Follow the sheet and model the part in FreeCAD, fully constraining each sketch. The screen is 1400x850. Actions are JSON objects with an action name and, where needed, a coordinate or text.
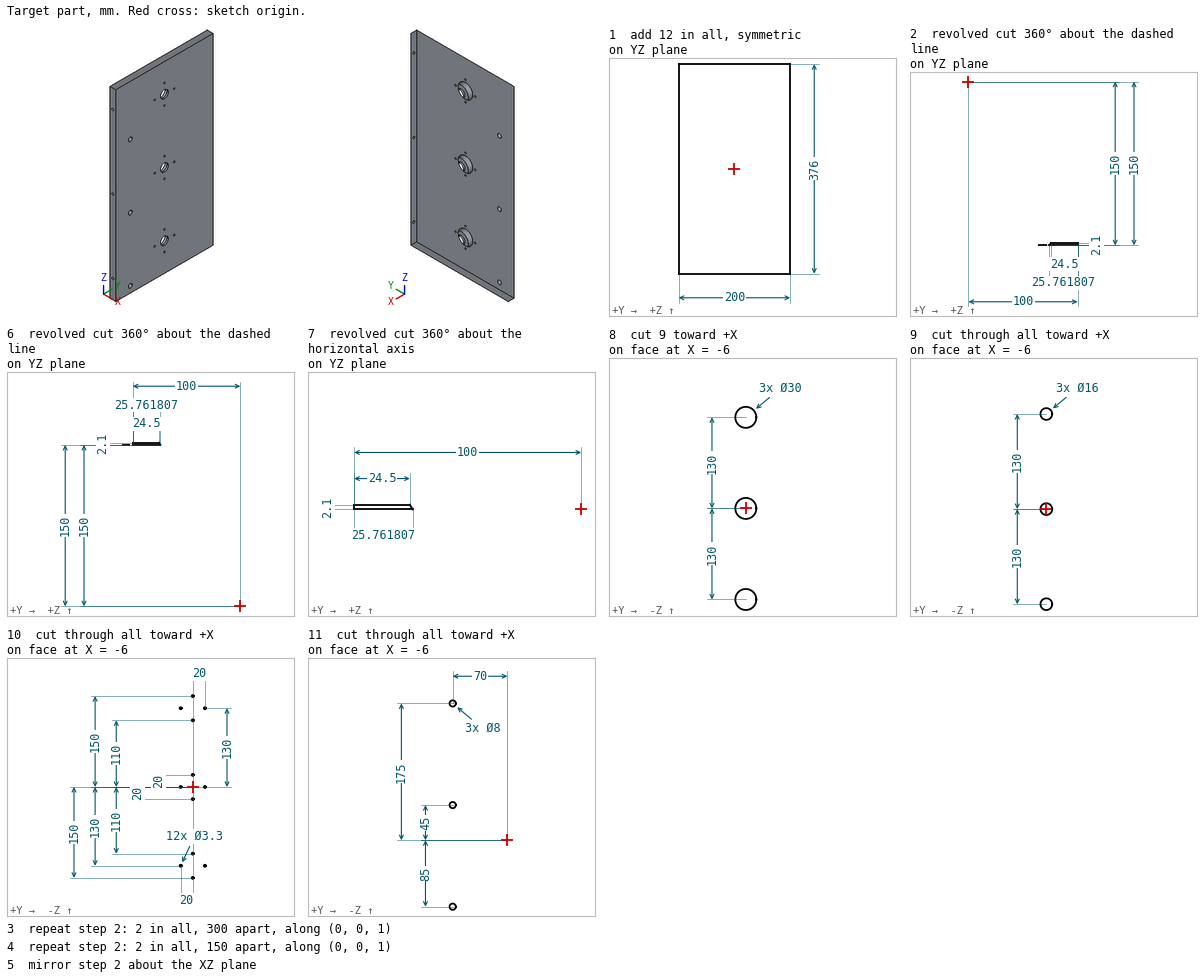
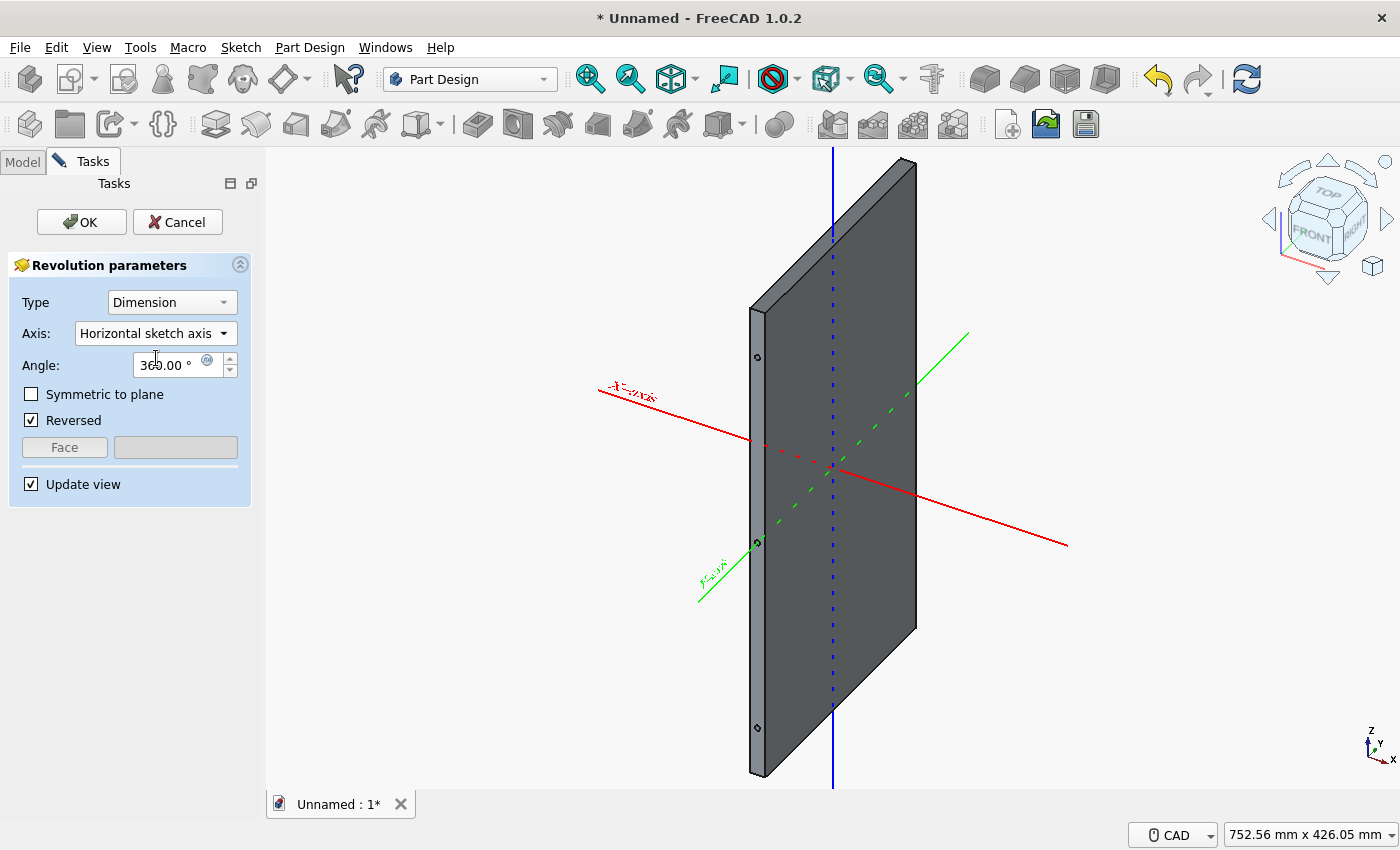
{"action": "left_click", "coordinate": [82, 222]}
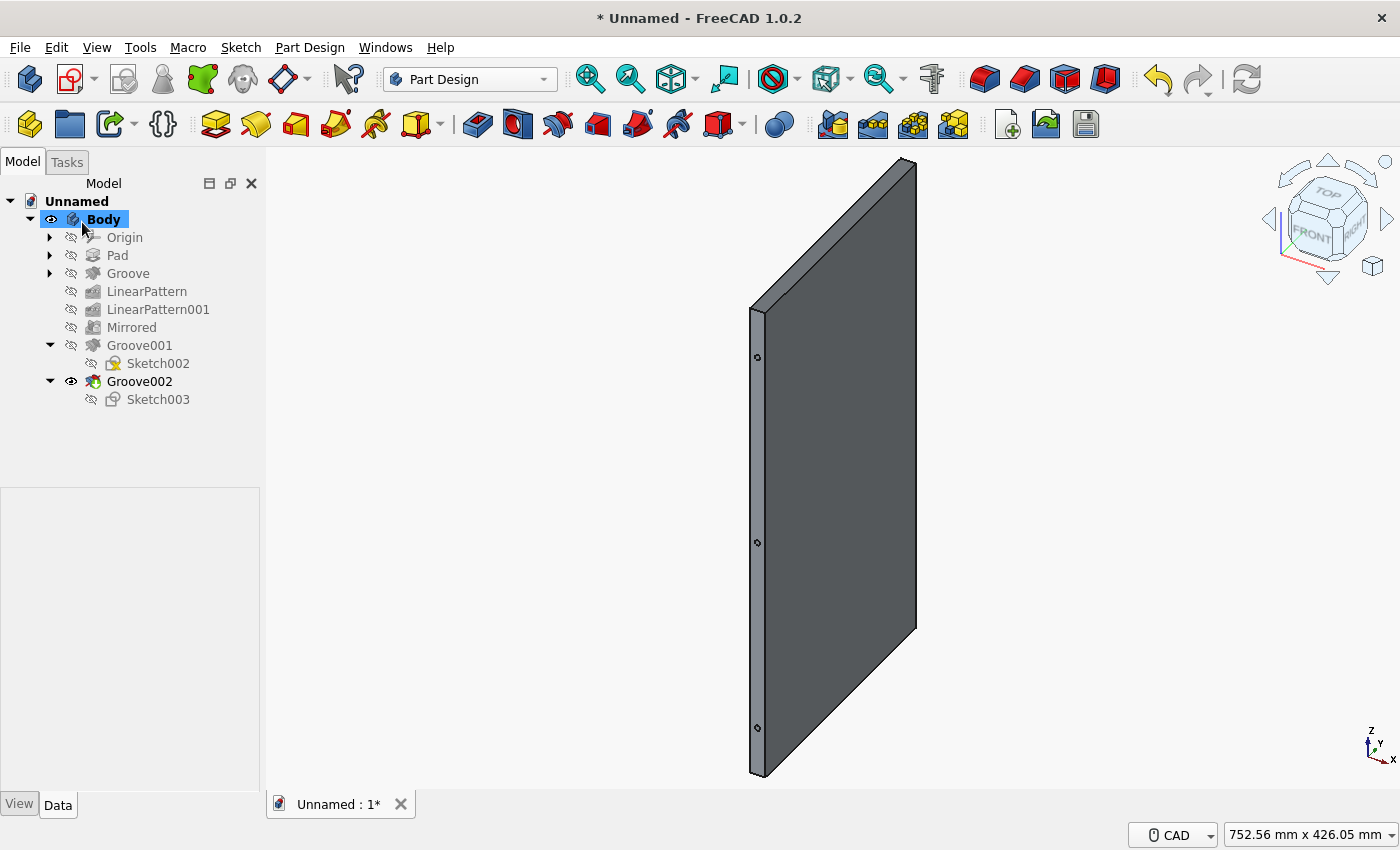
{"action": "key", "text": "6"}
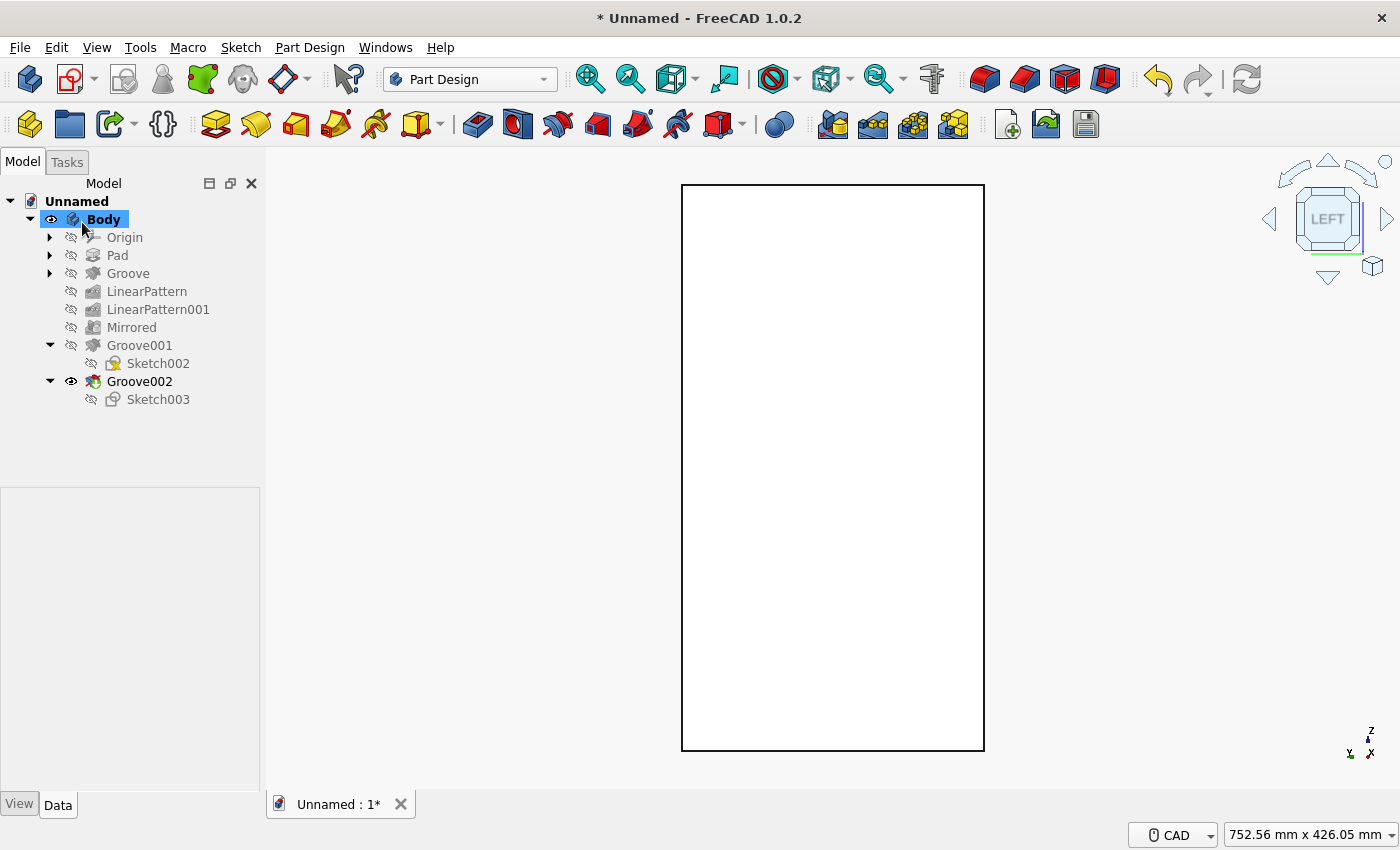
{"action": "left_click", "coordinate": [833, 467]}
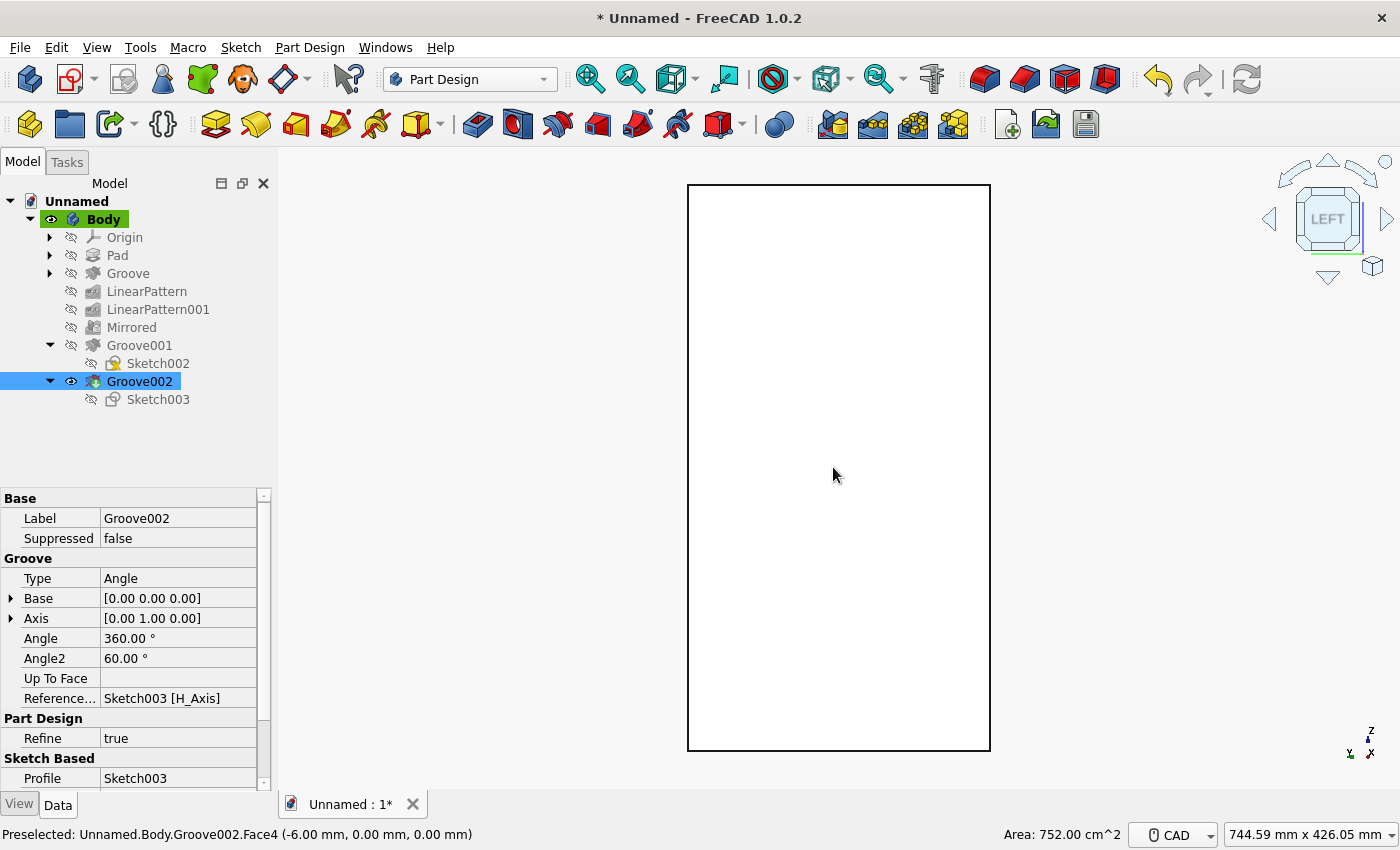
{"action": "left_click", "coordinate": [70, 80]}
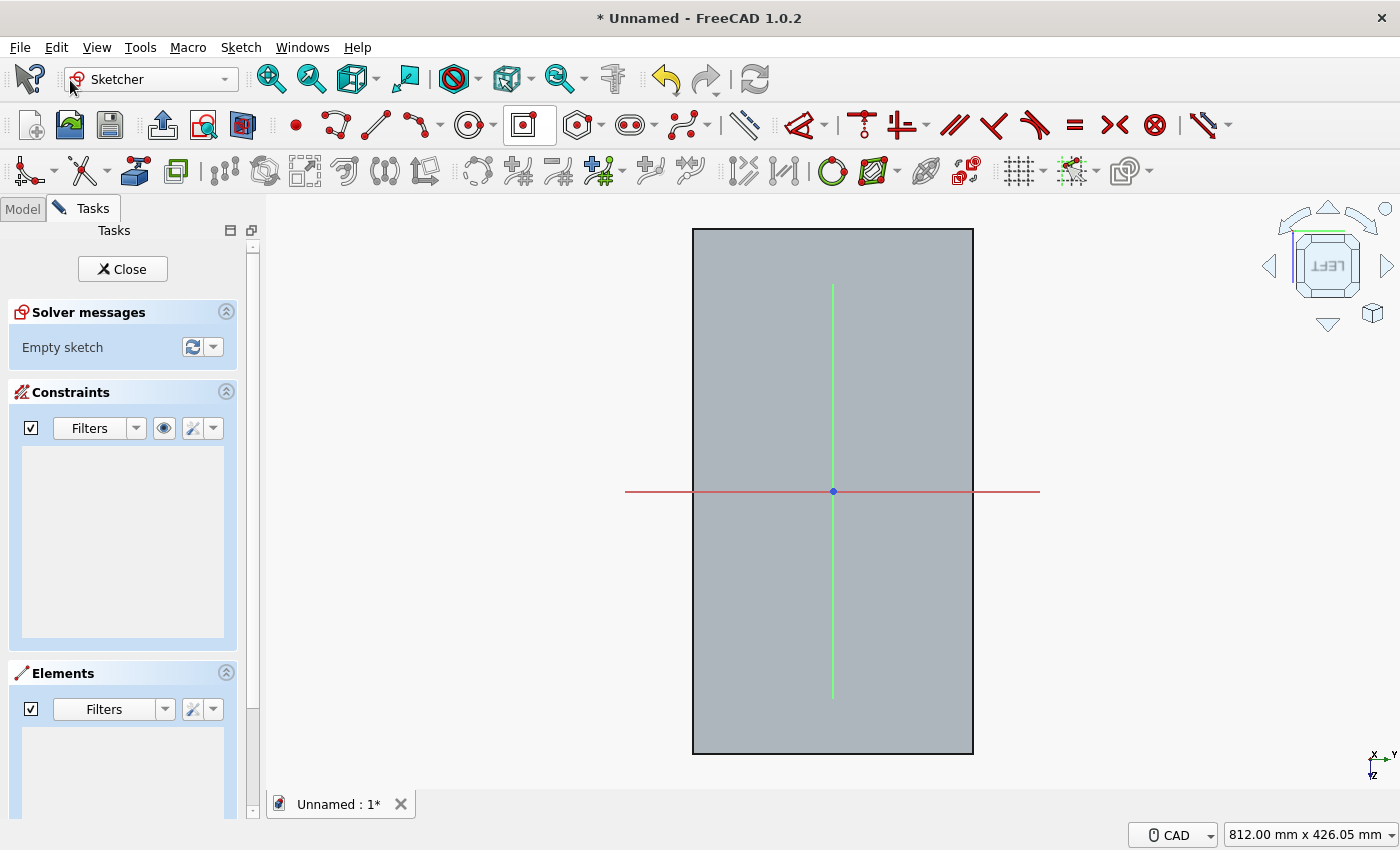
{"action": "left_click", "coordinate": [470, 126]}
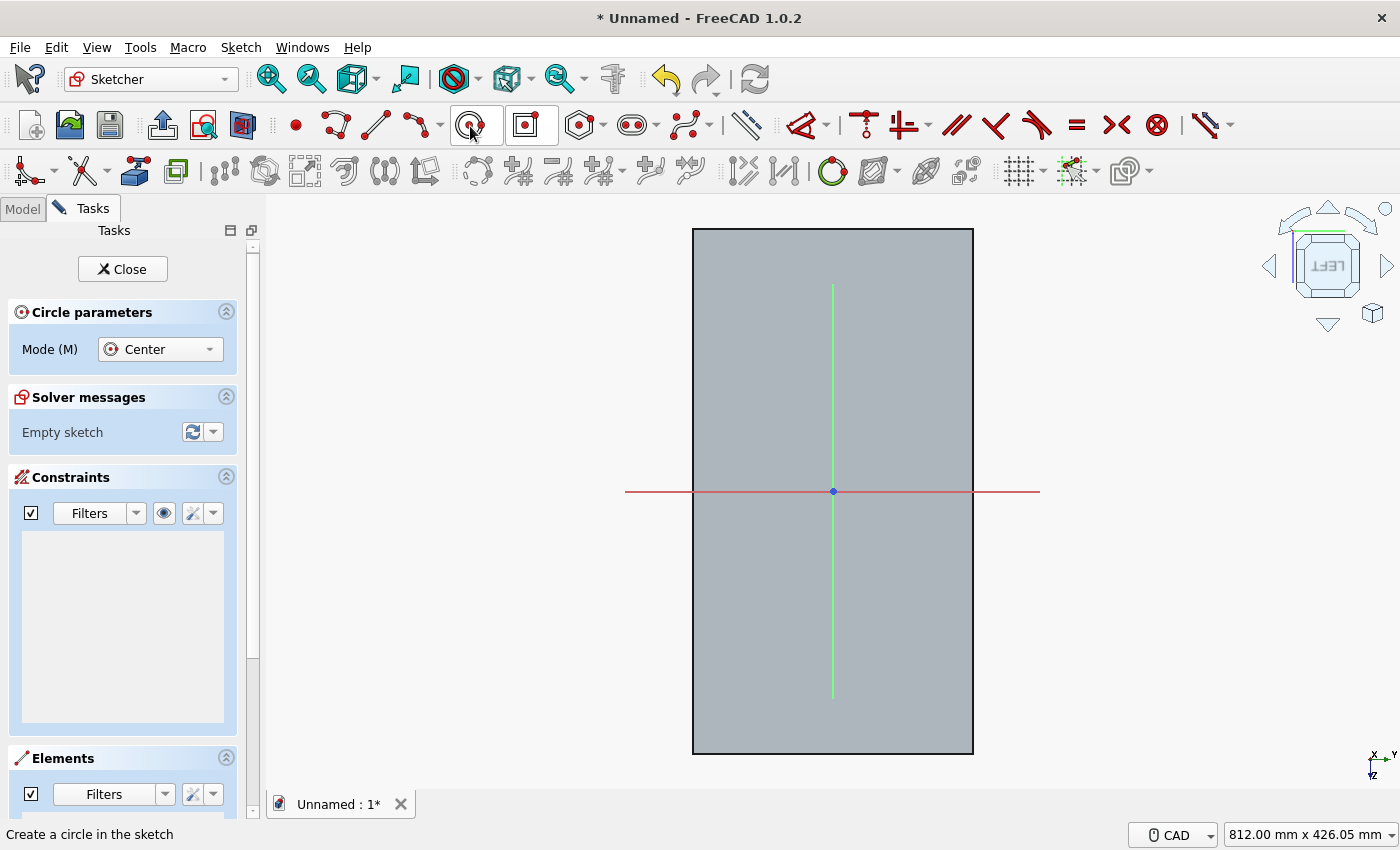
{"action": "left_click", "coordinate": [833, 310]}
{"action": "mouse_move", "coordinate": [848, 295]}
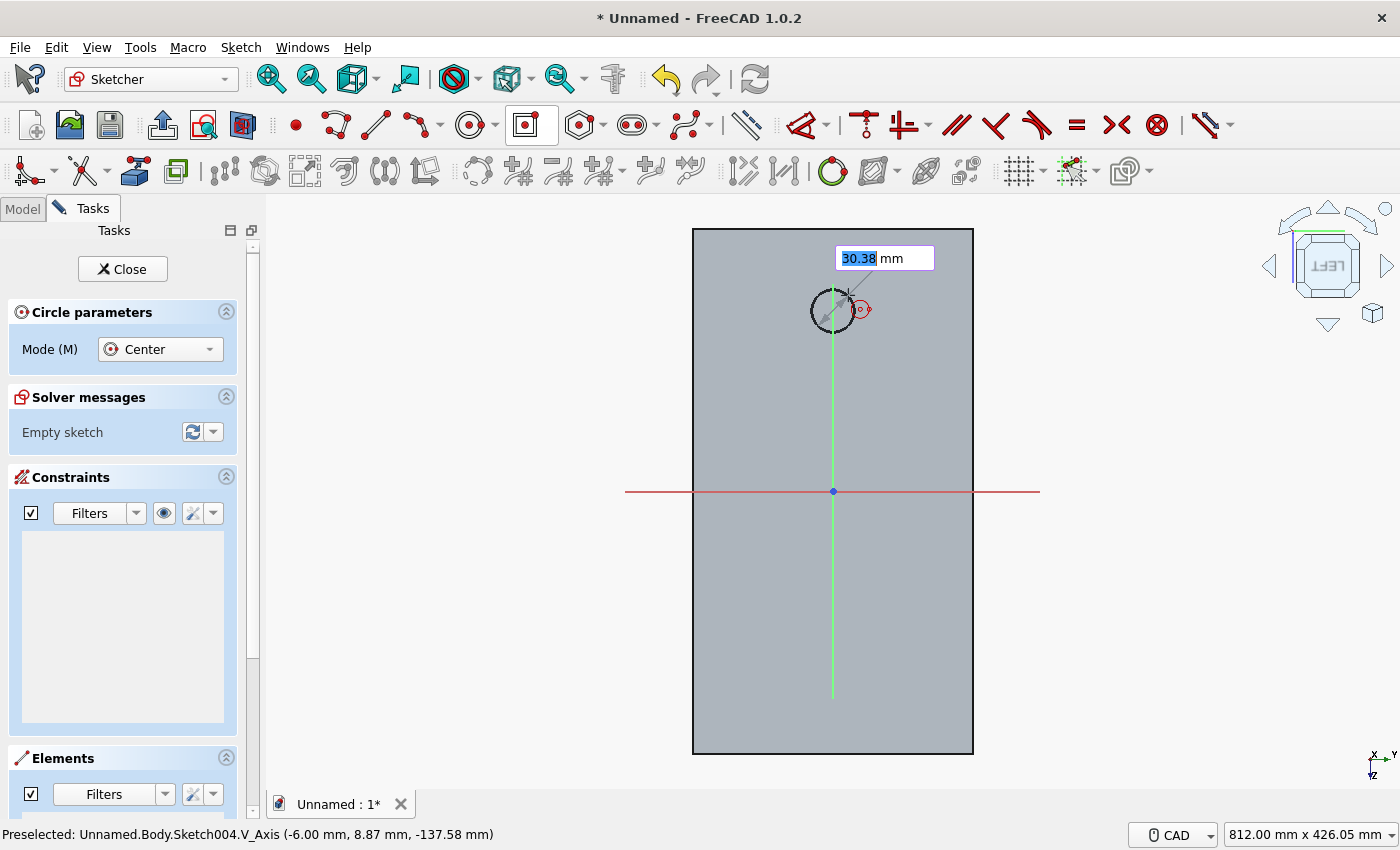
{"action": "type", "text": "30"}
{"action": "key", "text": "Return"}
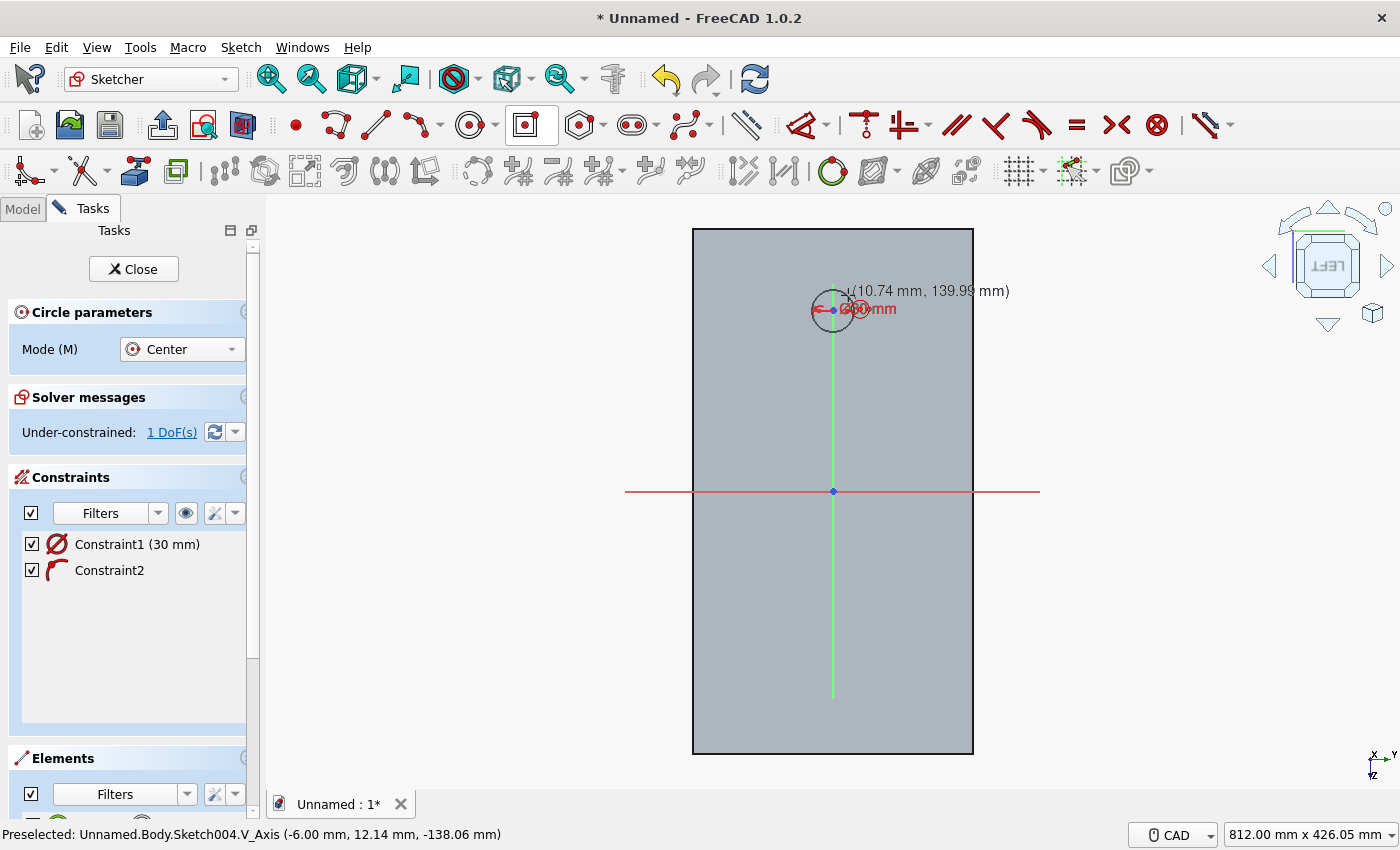
{"action": "left_click", "coordinate": [833, 492]}
{"action": "mouse_move", "coordinate": [848, 477]}